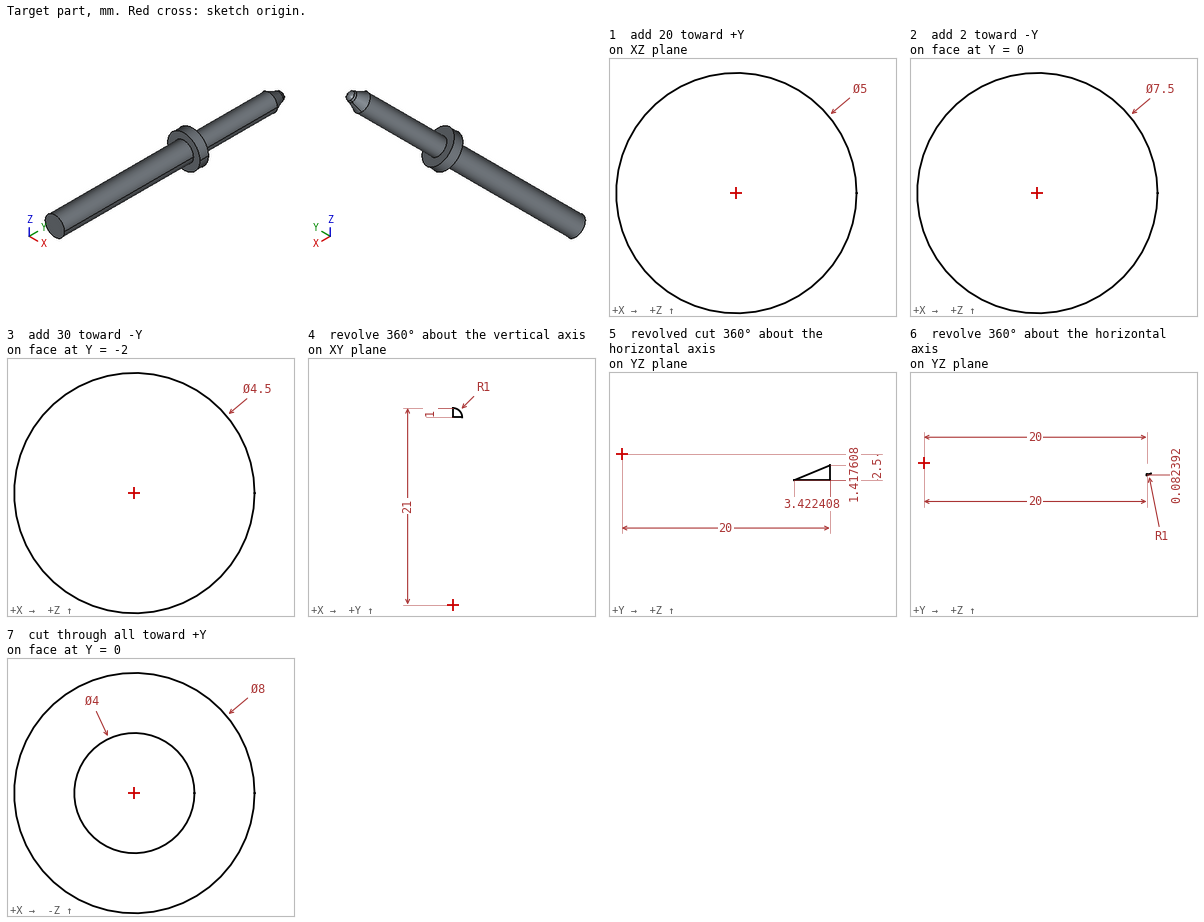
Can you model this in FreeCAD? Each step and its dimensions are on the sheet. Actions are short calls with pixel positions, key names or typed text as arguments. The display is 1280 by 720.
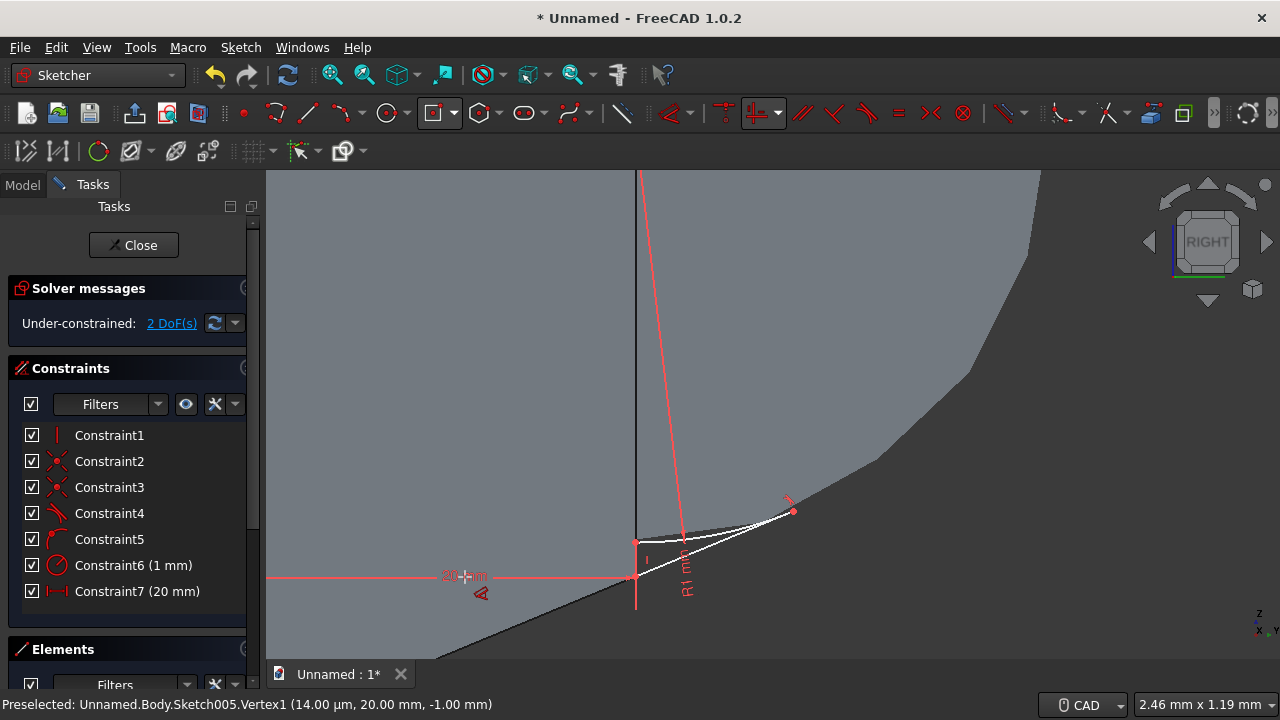
scroll(718, 586, up, 7)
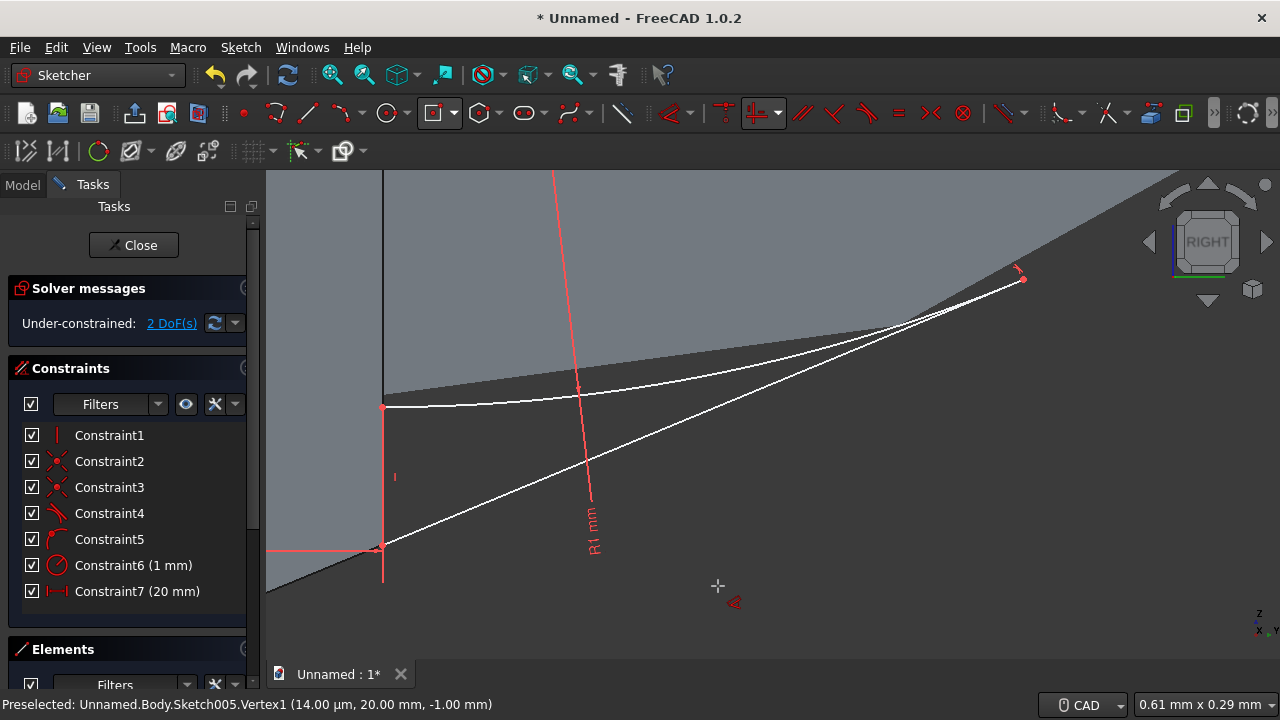
scroll(705, 568, down, 9)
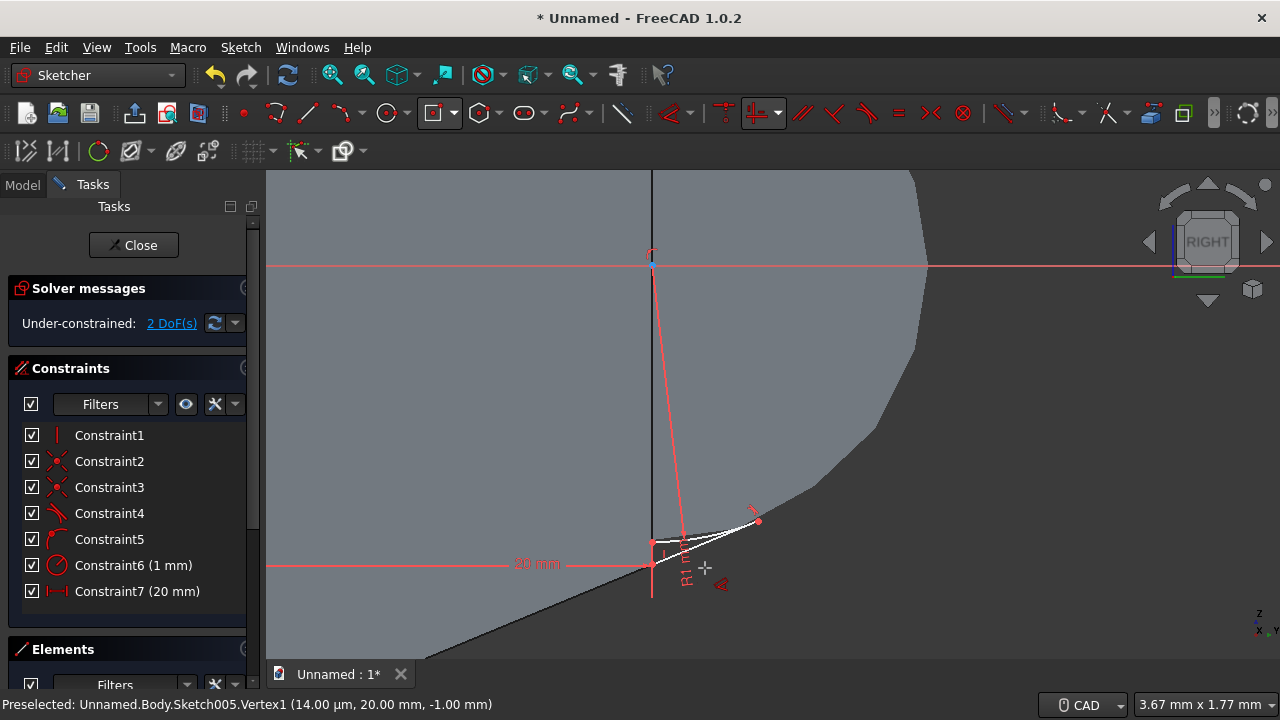
click(652, 266)
click(473, 232)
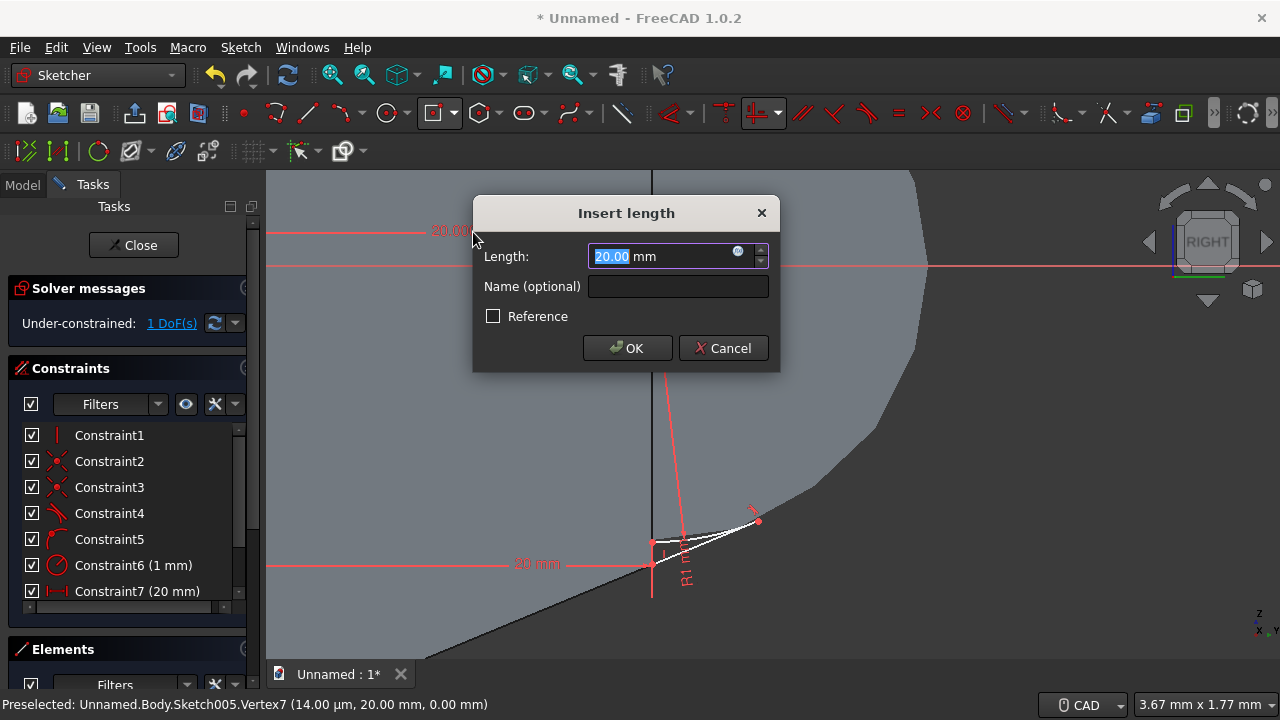
text(20)
key(Return)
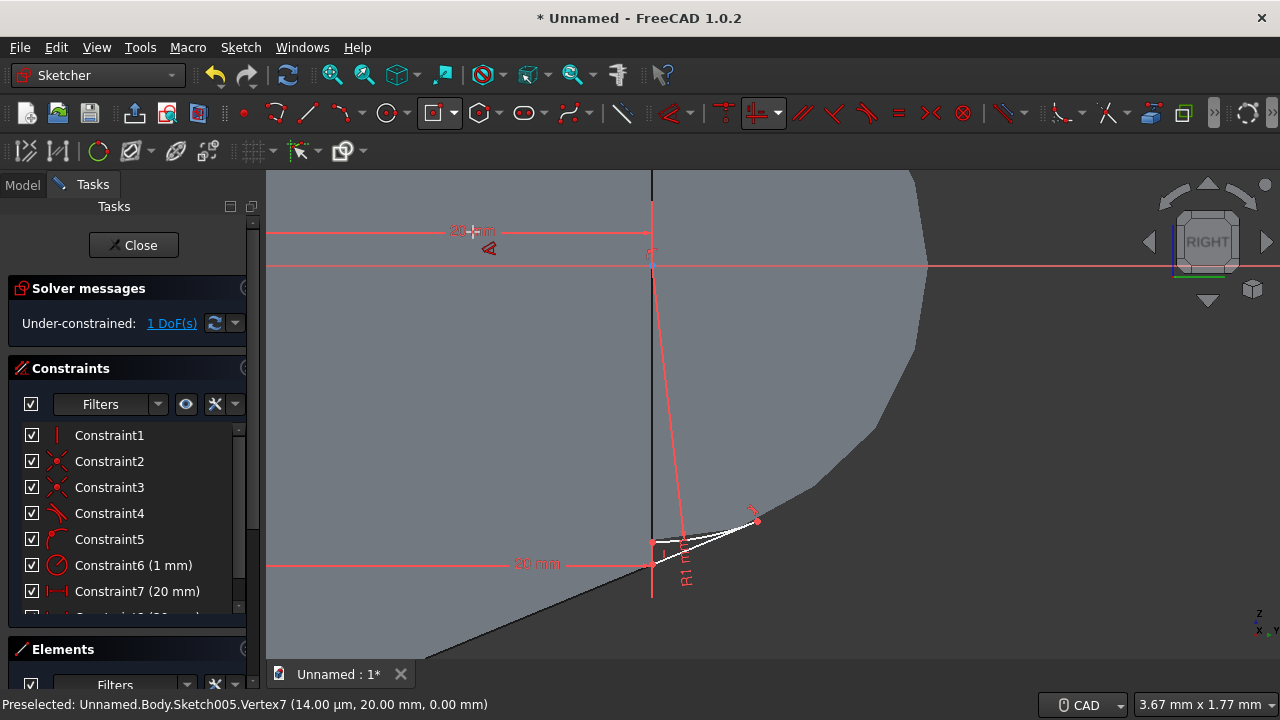
scroll(652, 551, up, 3)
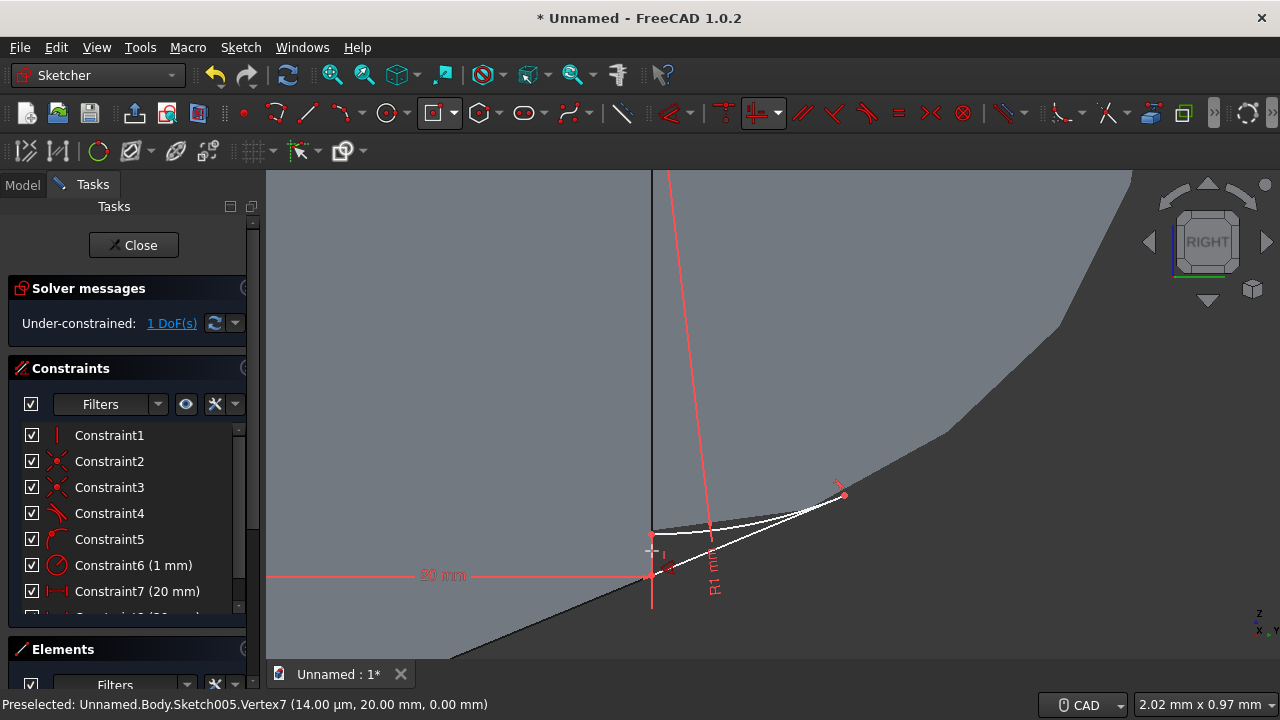
click(652, 551)
click(618, 555)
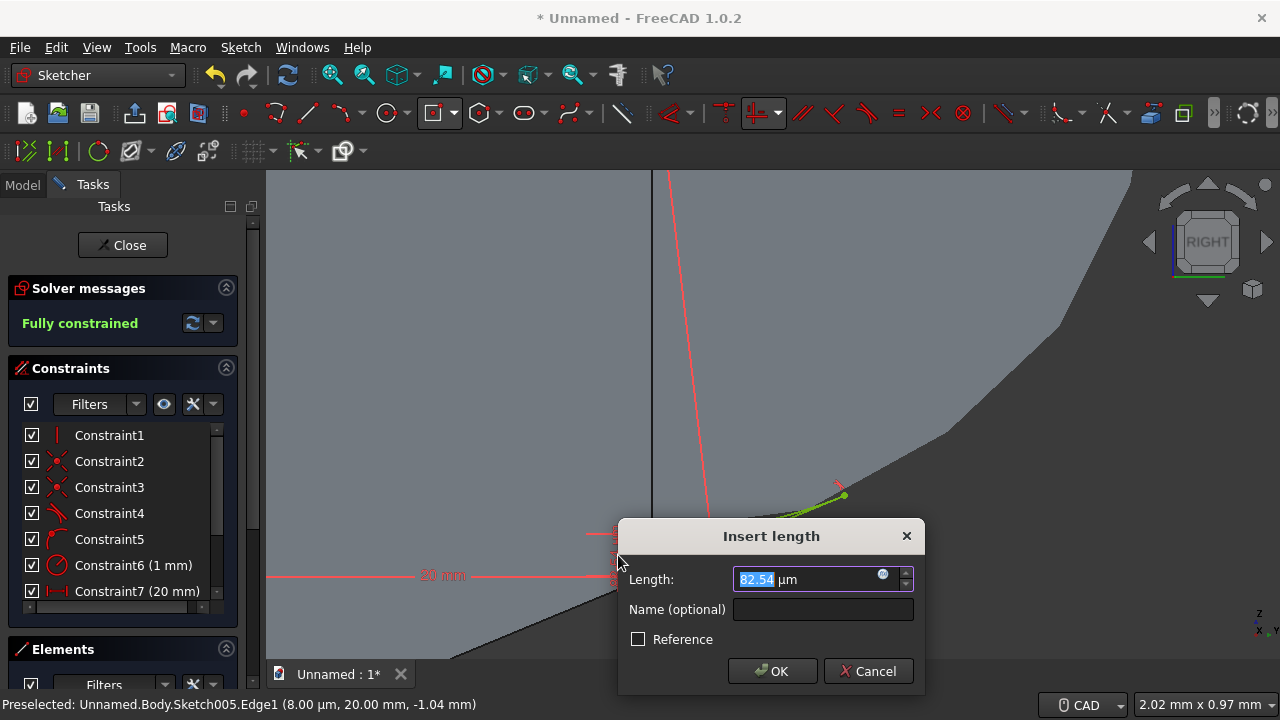
key(ctrl+a)
text(0.082392 mm)
key(Return)
key(Escape)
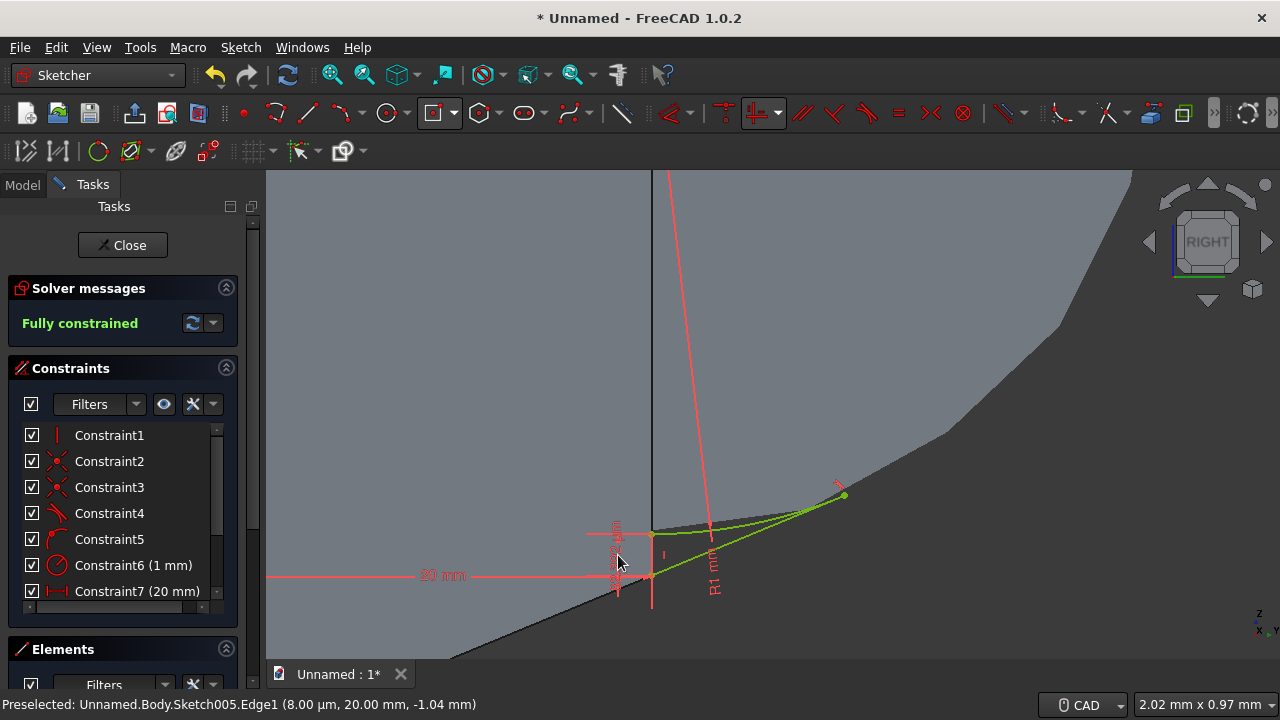
click(123, 245)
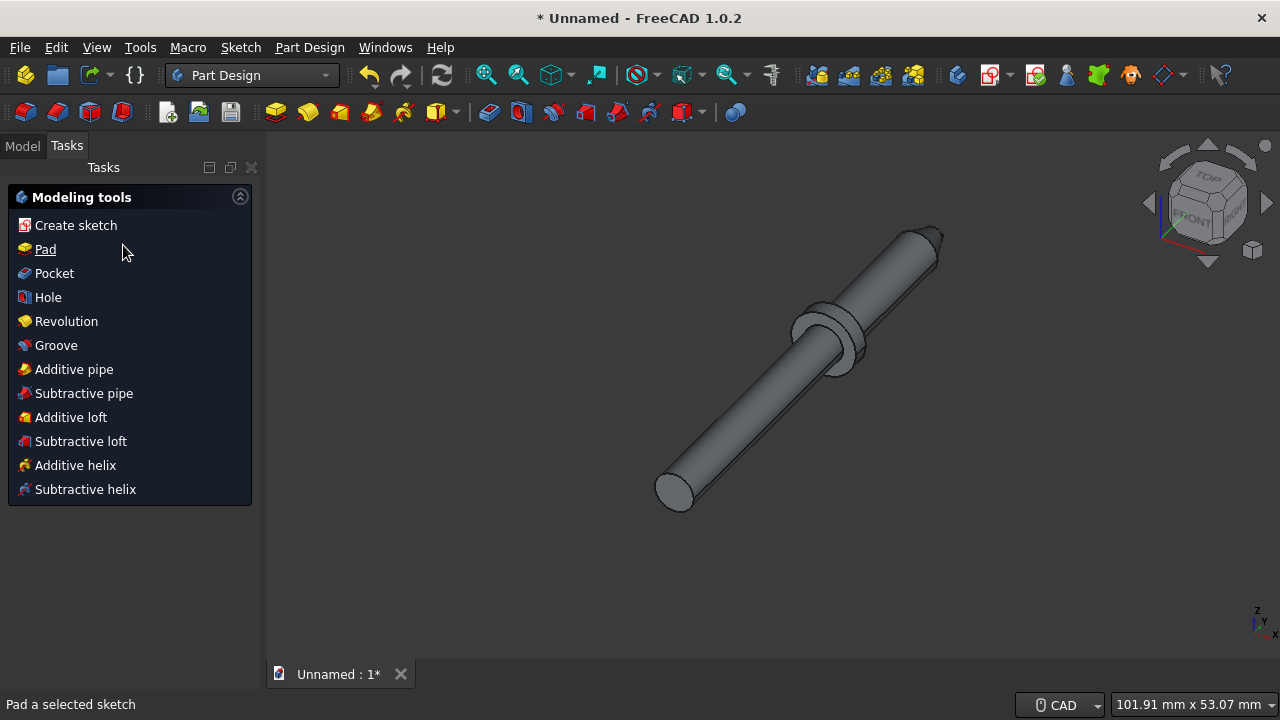
click(308, 112)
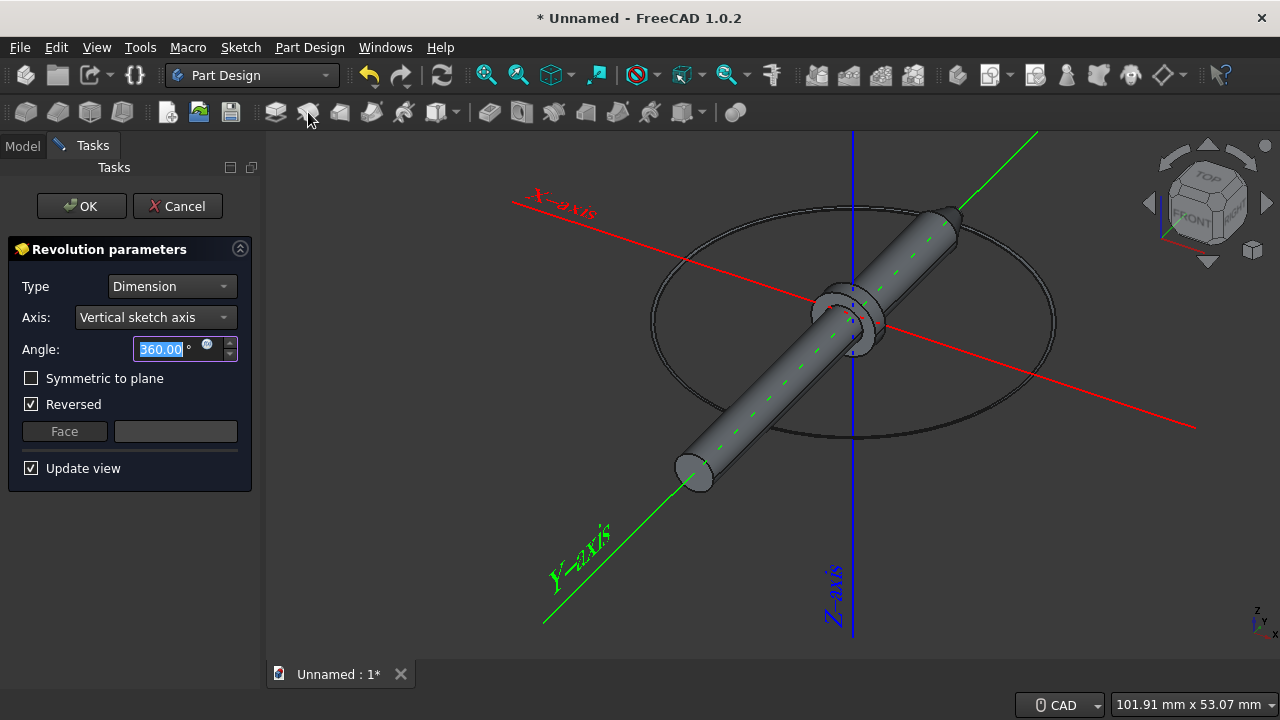
click(156, 318)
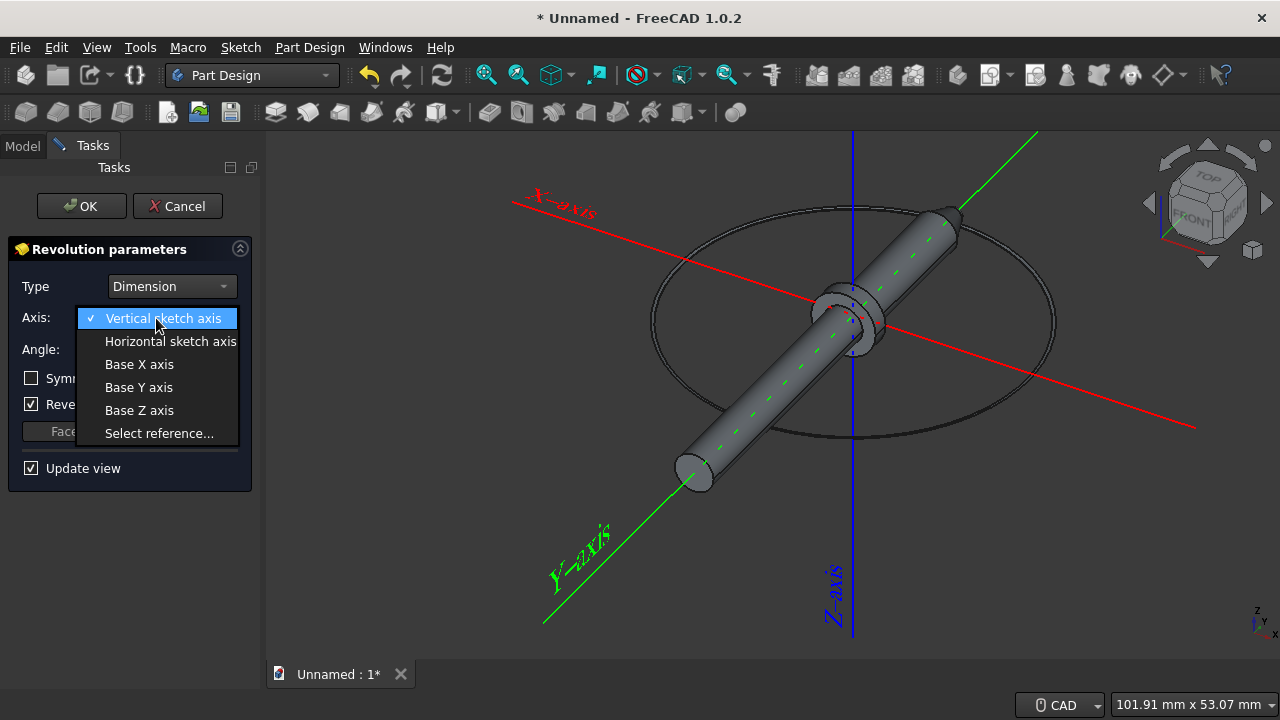
click(156, 342)